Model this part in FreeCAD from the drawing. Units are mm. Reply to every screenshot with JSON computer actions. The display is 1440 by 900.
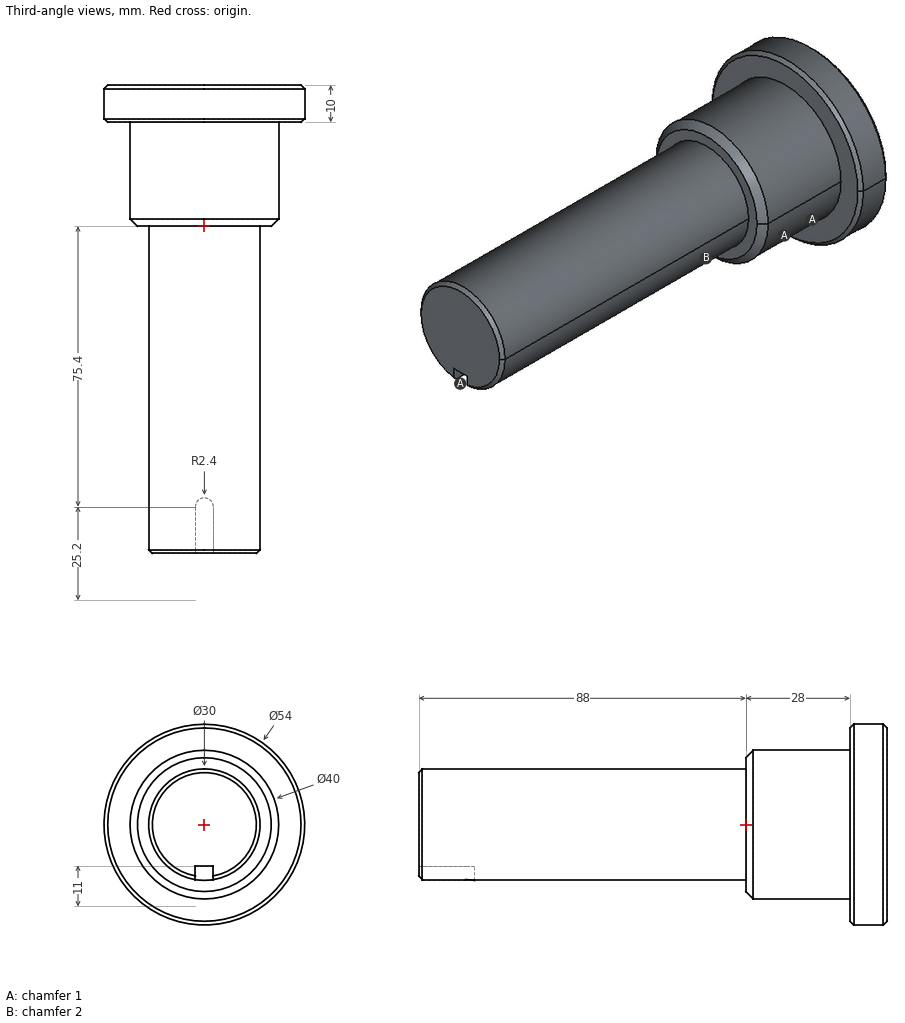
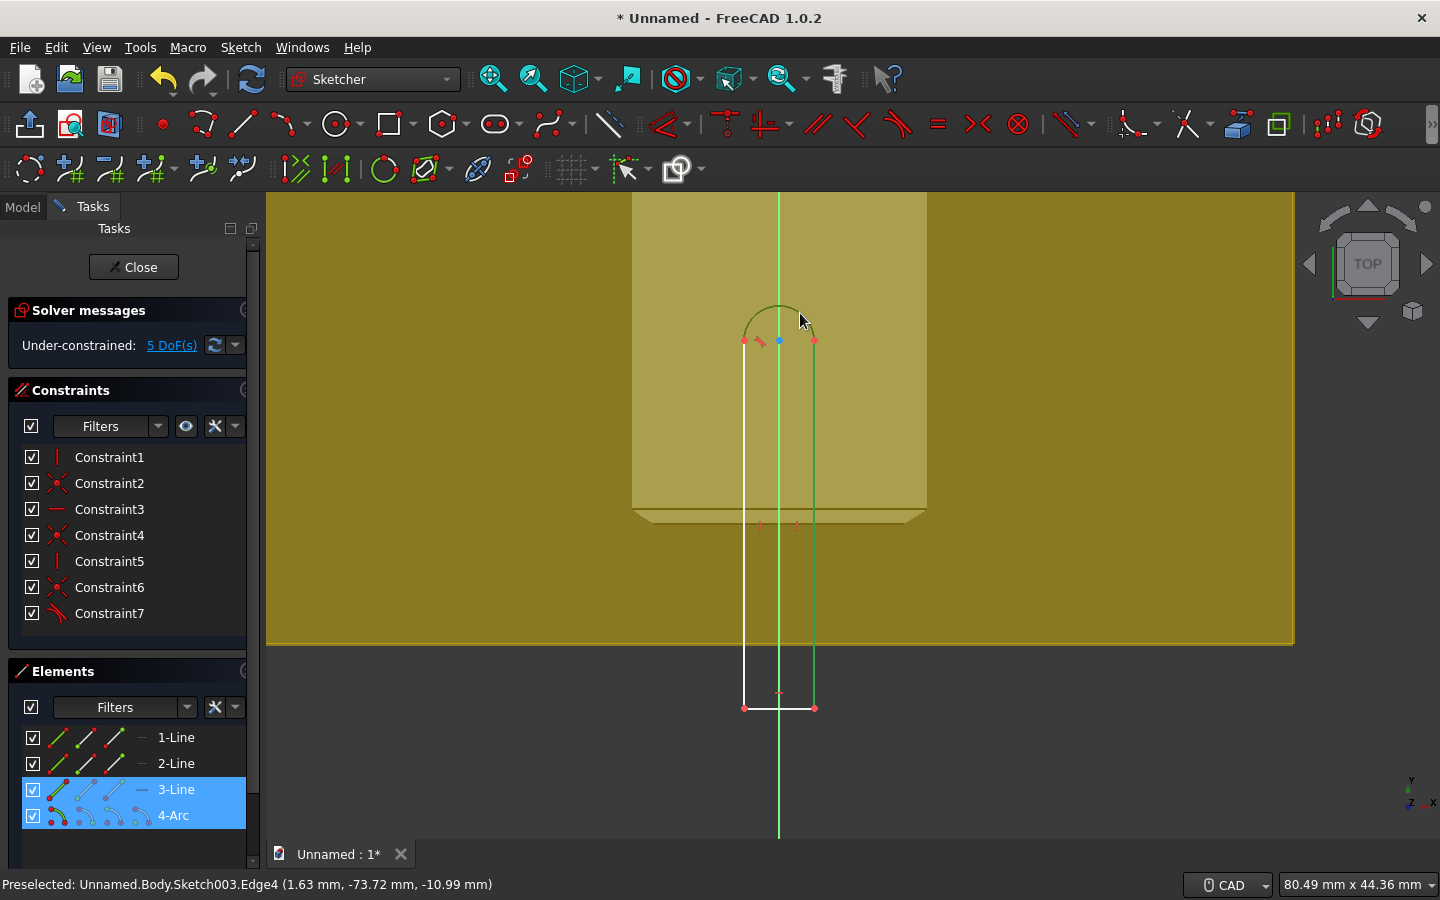
{"action": "left_click", "coordinate": [898, 124]}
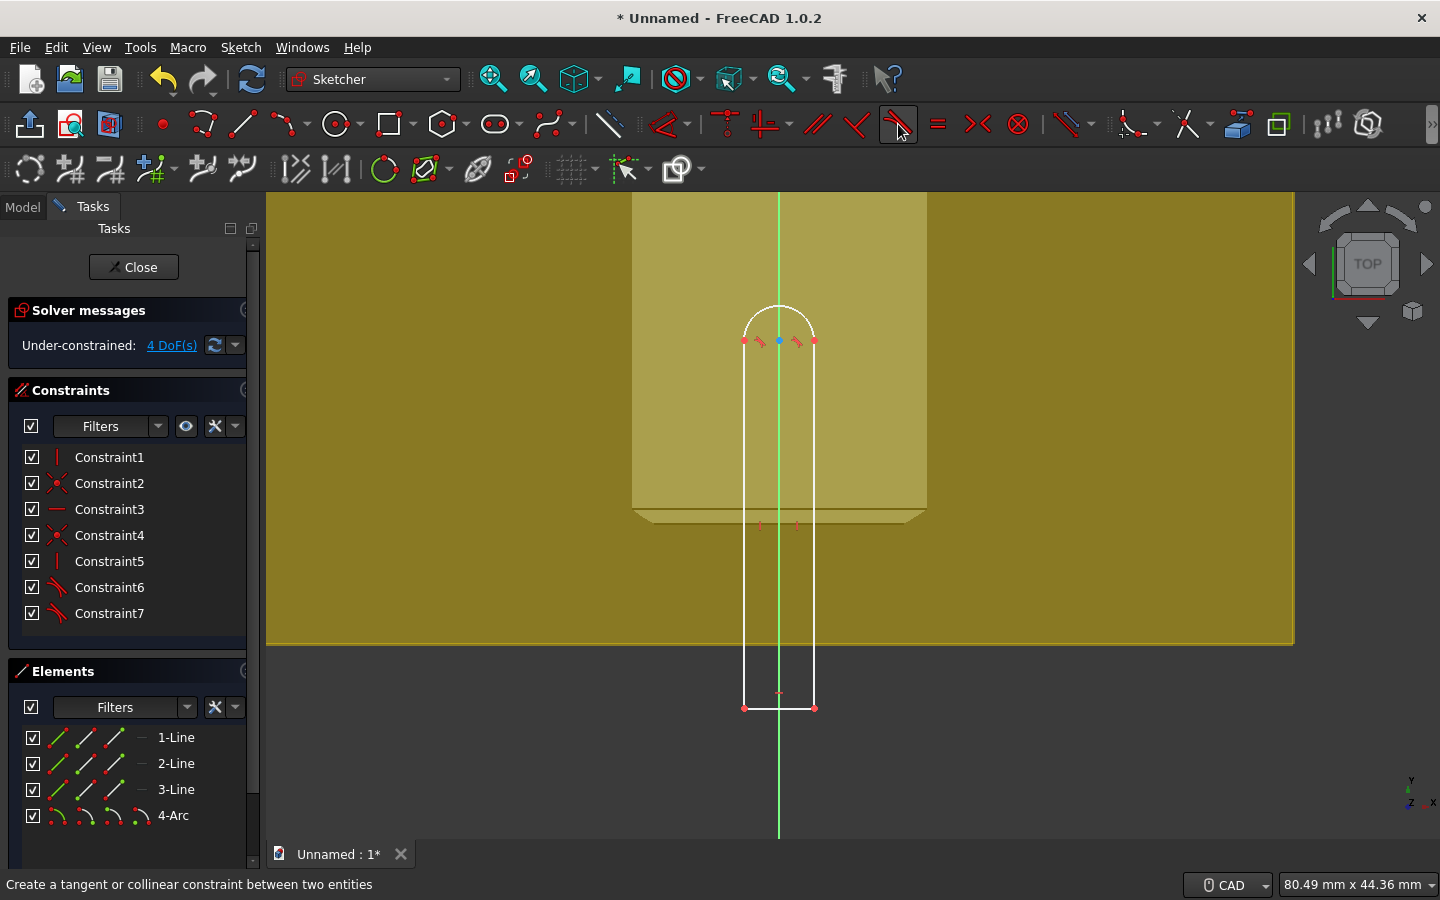
{"action": "left_click", "coordinate": [779, 341]}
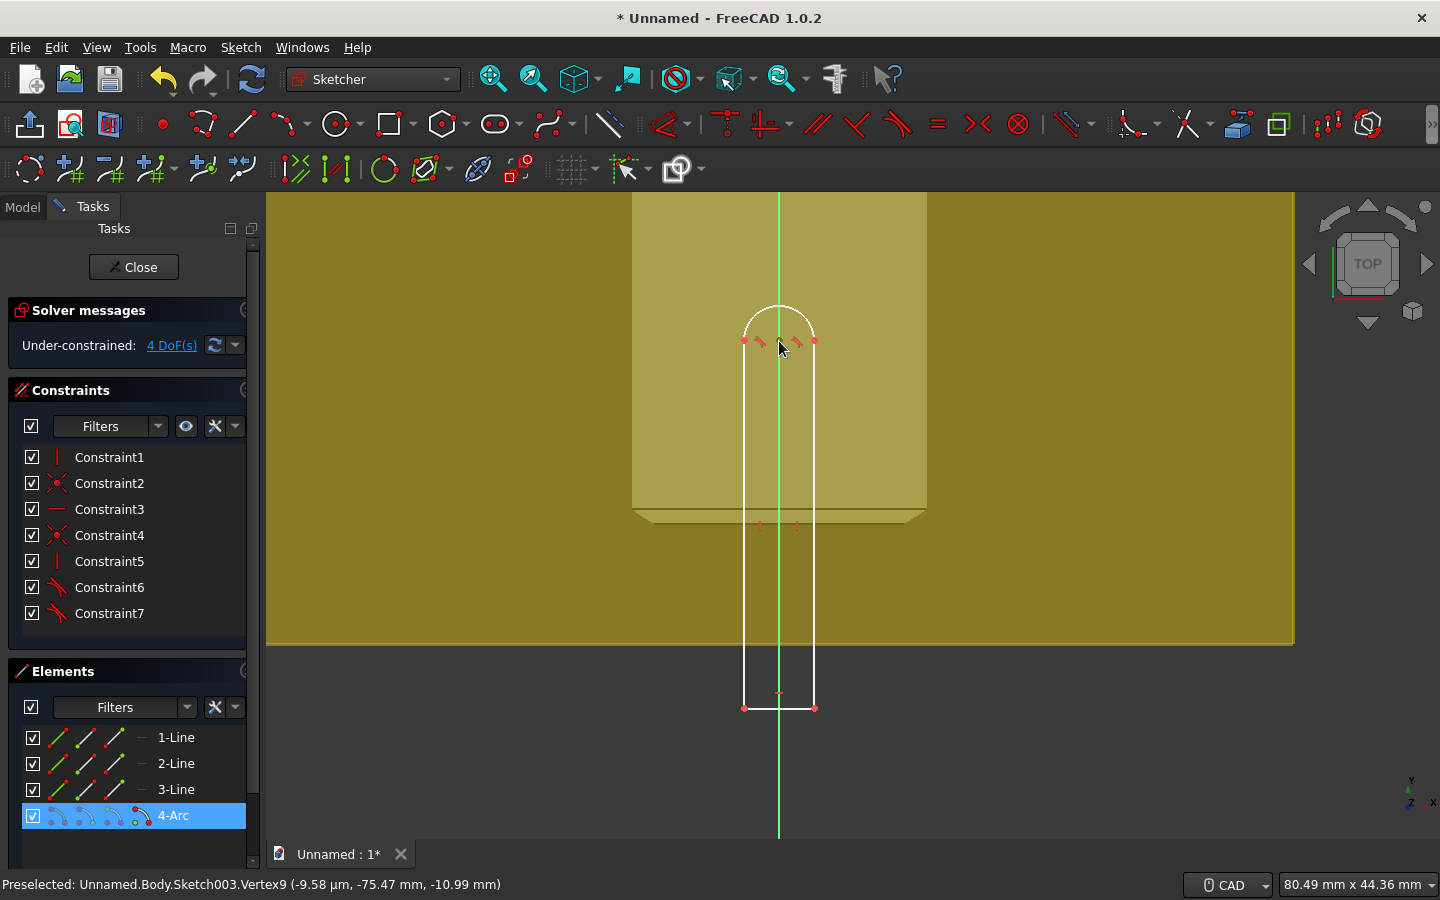
{"action": "left_click", "coordinate": [779, 769]}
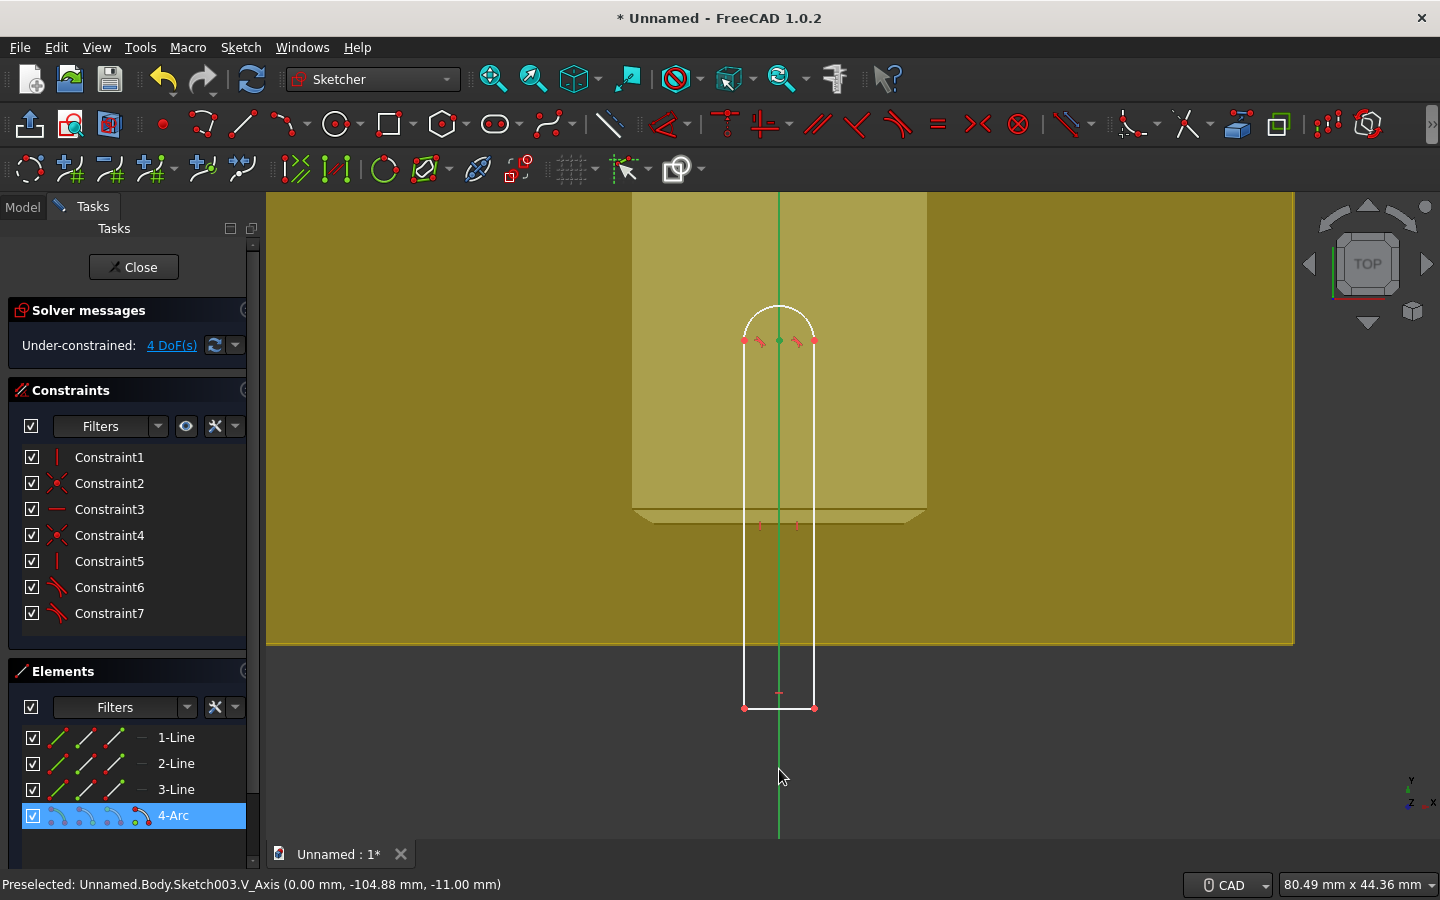
{"action": "key", "text": "c"}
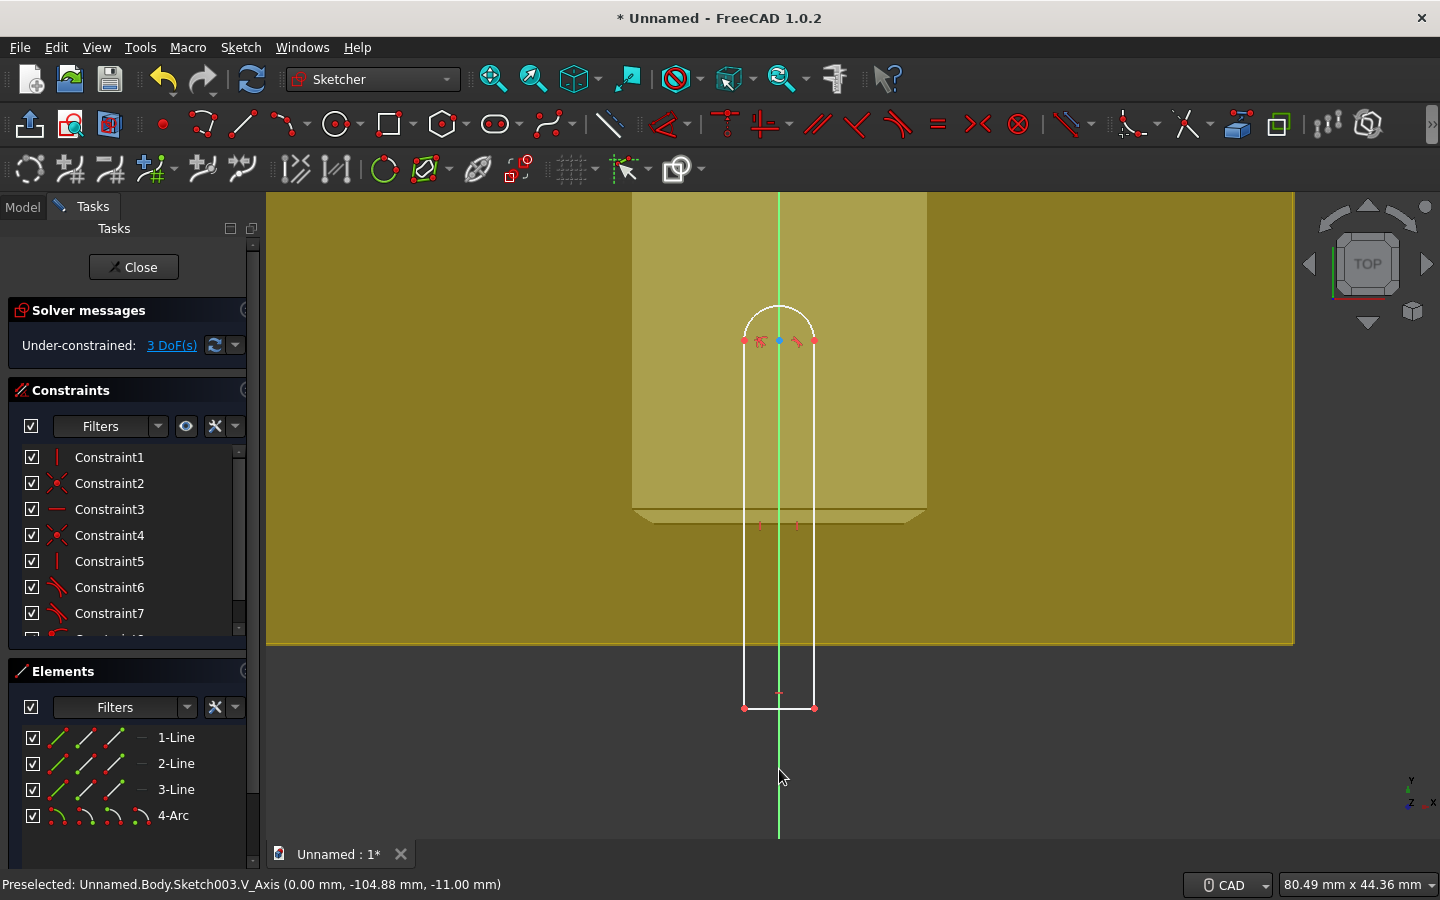
{"action": "left_click", "coordinate": [800, 313]}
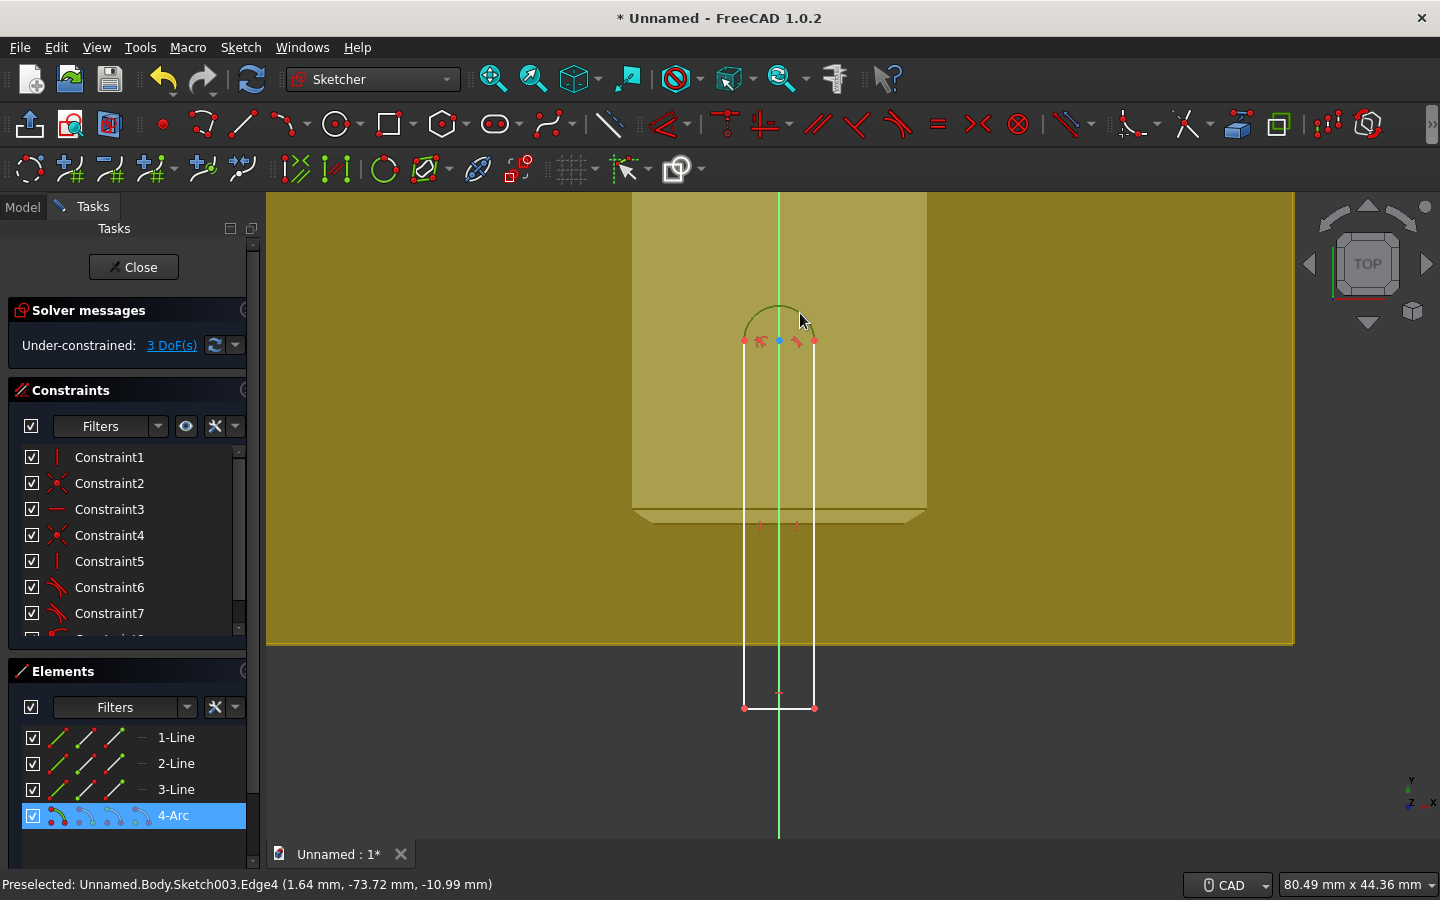
{"action": "left_click", "coordinate": [690, 124]}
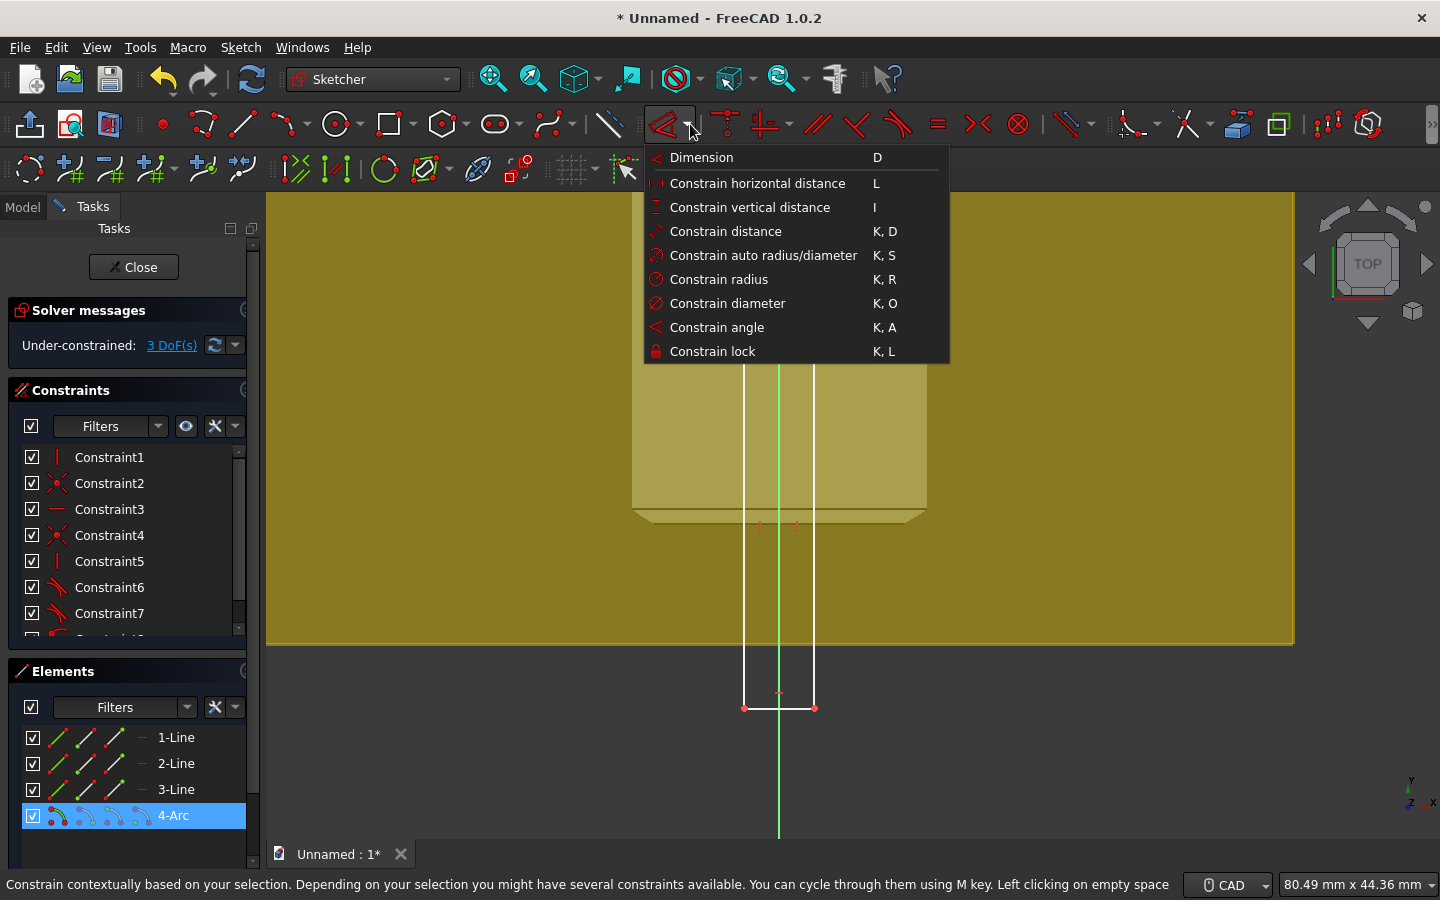
{"action": "left_click", "coordinate": [797, 279]}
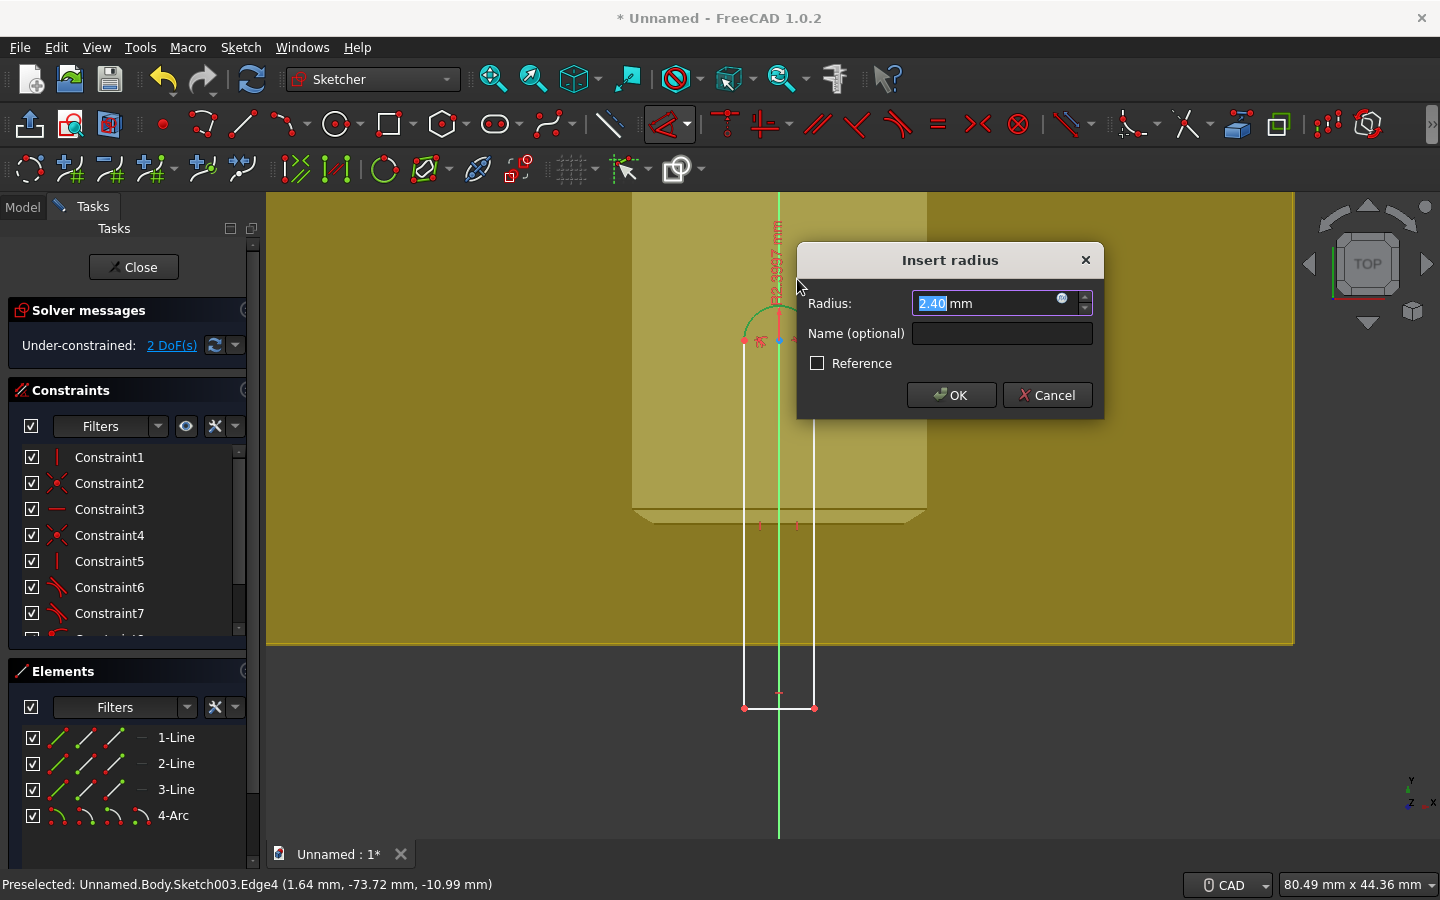
{"action": "type", "text": "2.4"}
{"action": "key", "text": "Return"}